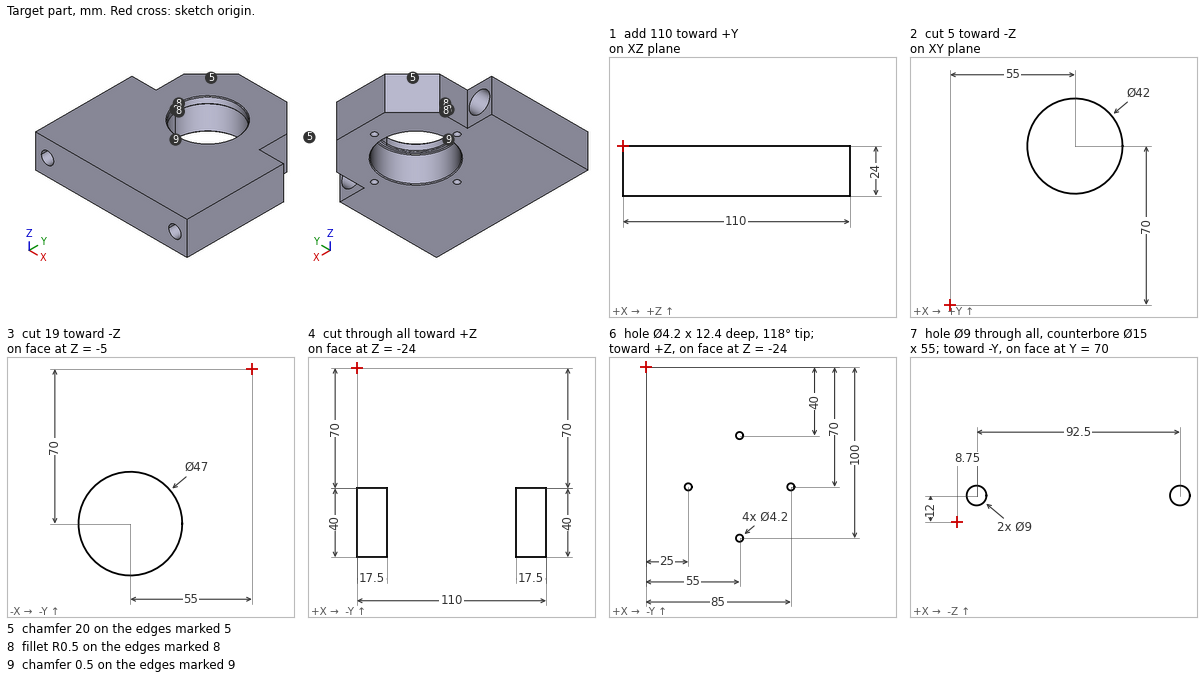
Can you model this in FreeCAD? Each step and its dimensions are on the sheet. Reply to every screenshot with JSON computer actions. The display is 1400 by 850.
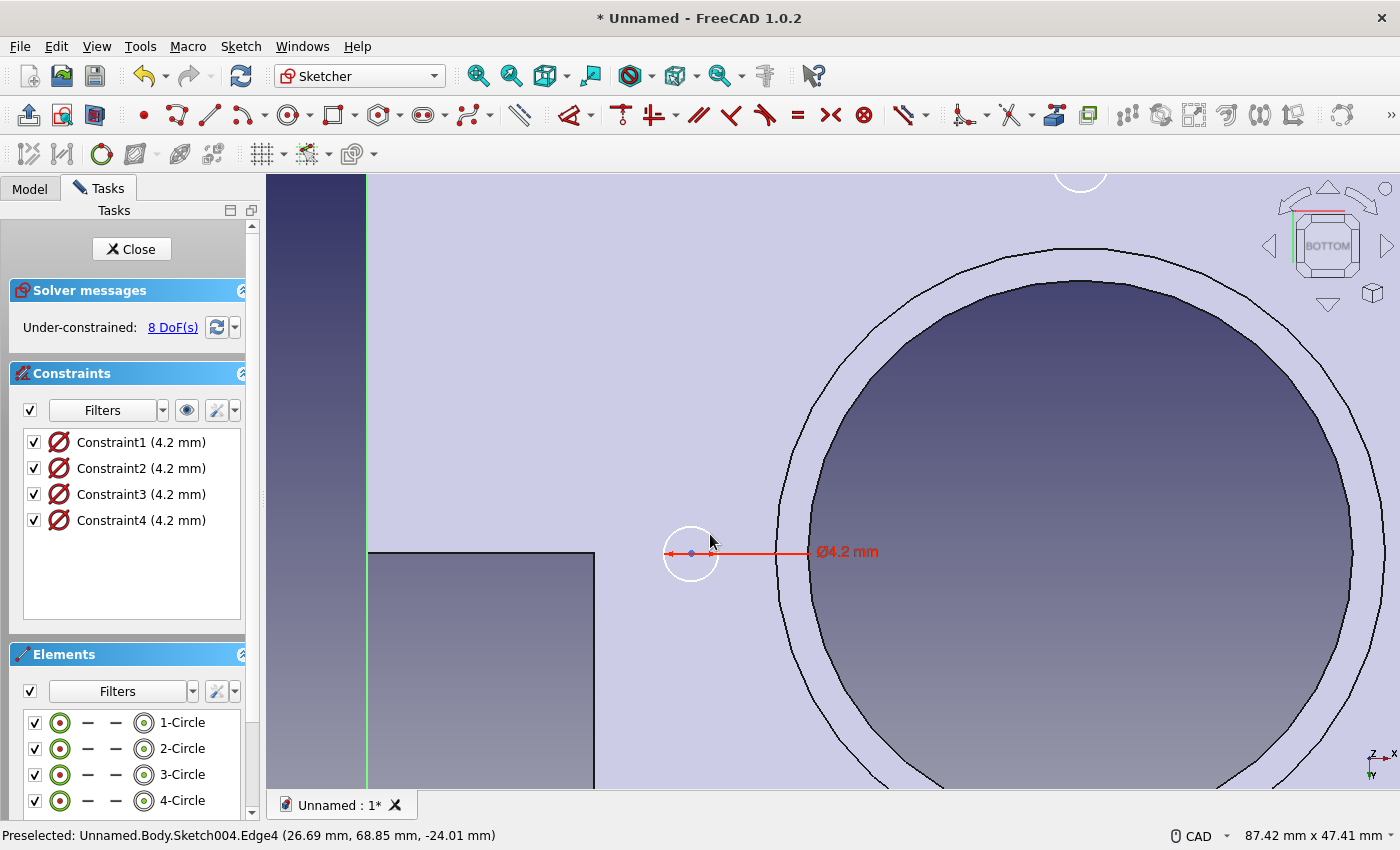
{"action": "scroll", "coordinate": [692, 557], "scroll_direction": "down", "scroll_amount": 6}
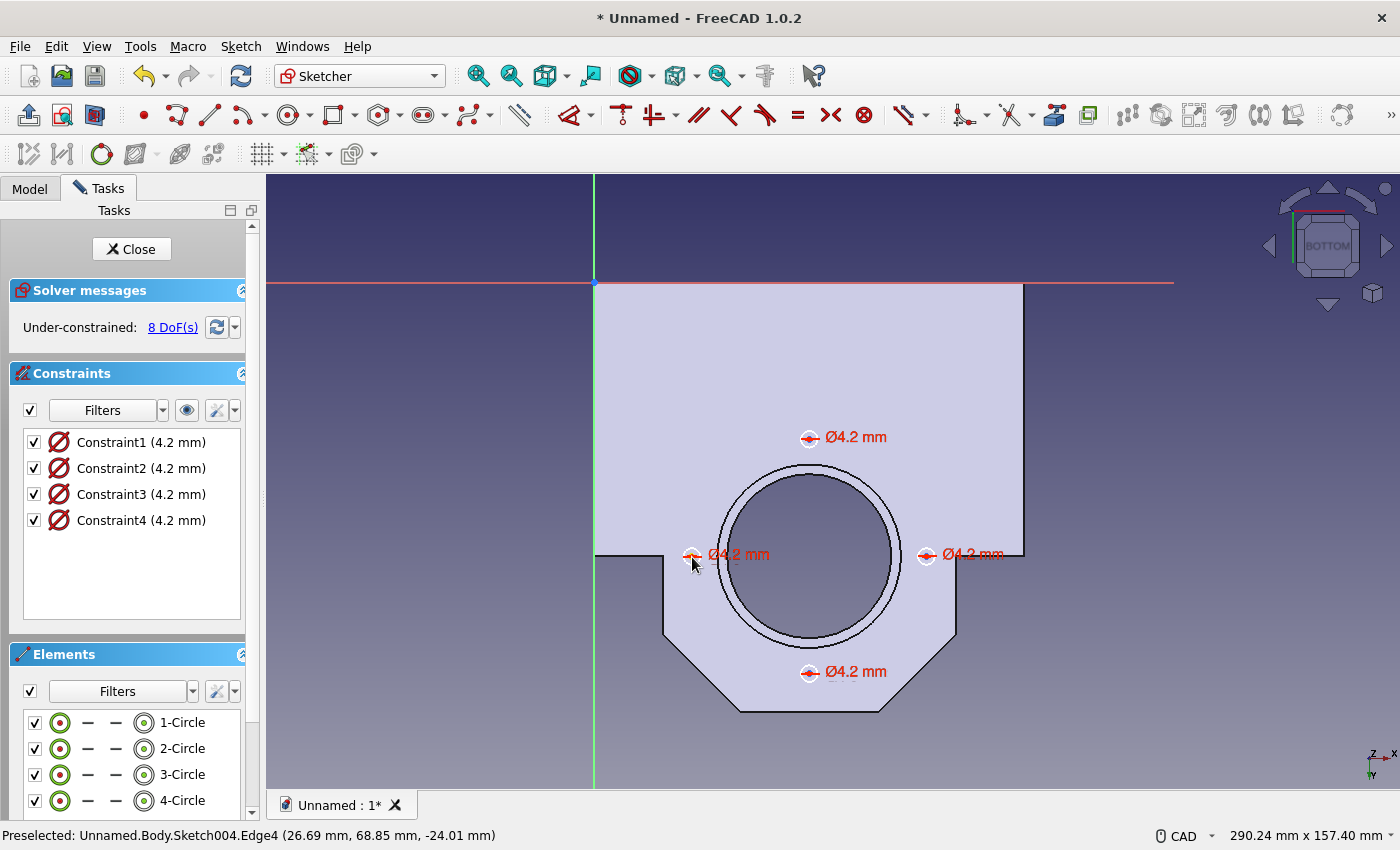
{"action": "left_click", "coordinate": [809, 674]}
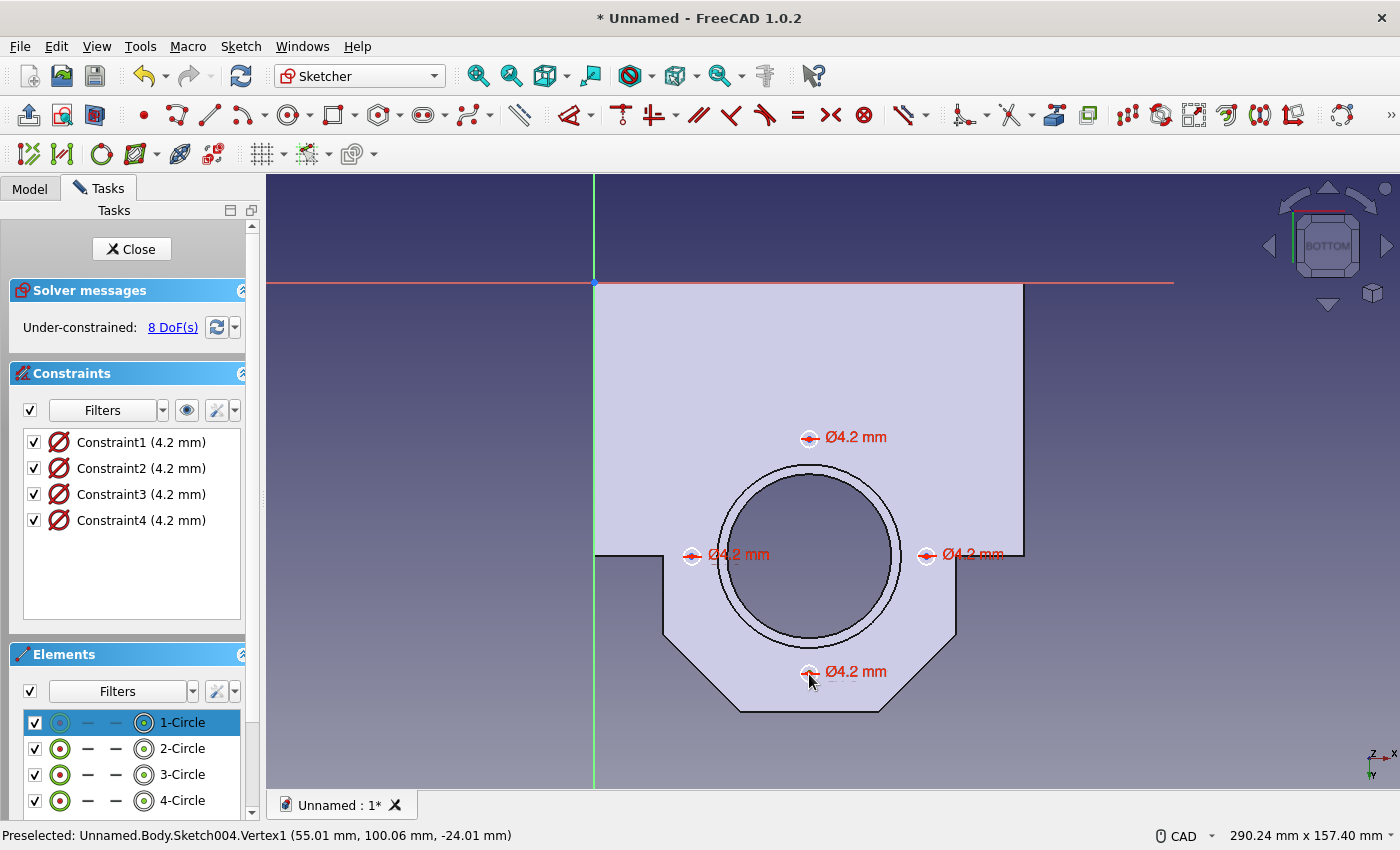
{"action": "left_click", "coordinate": [809, 439]}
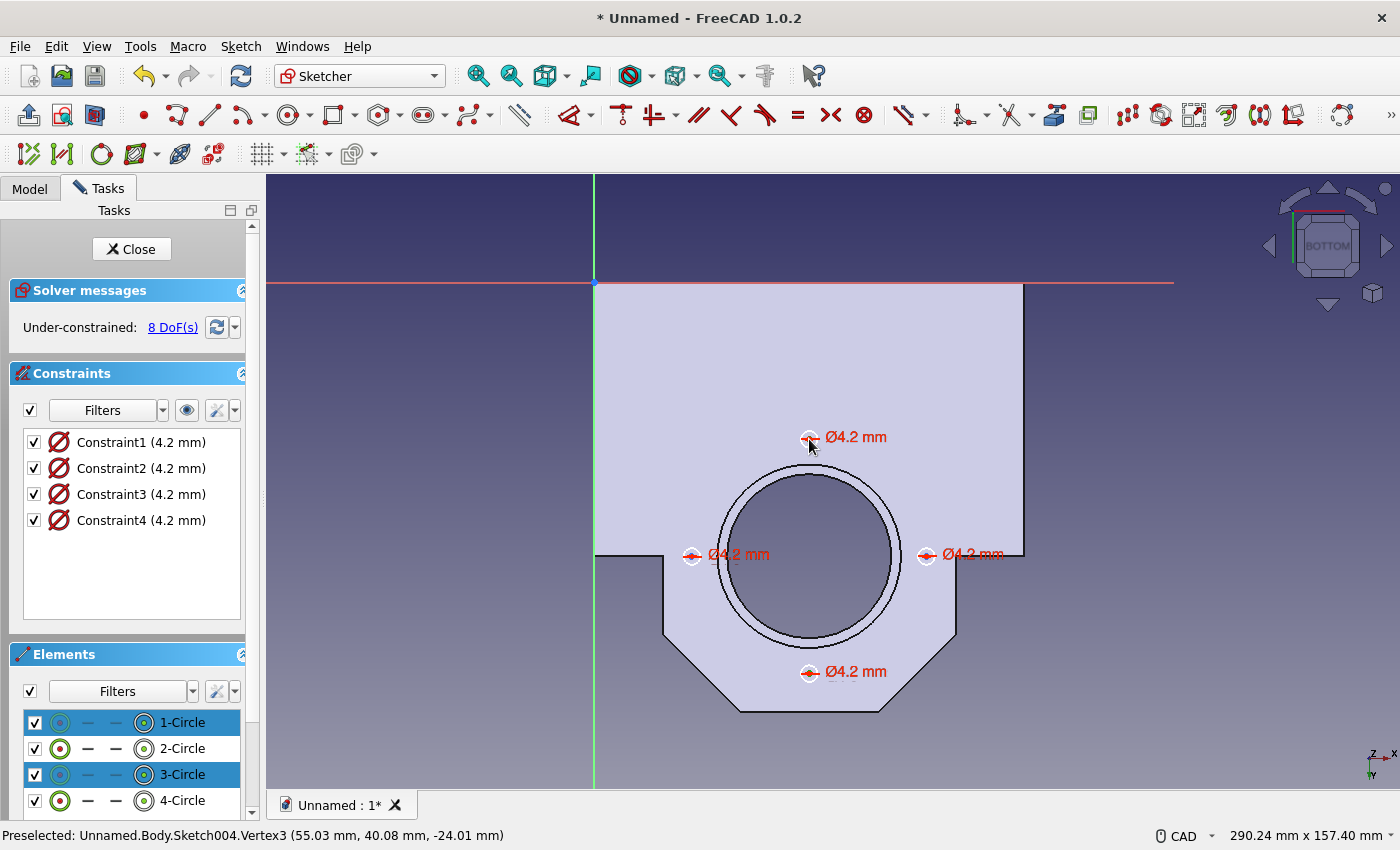
{"action": "key", "text": "v"}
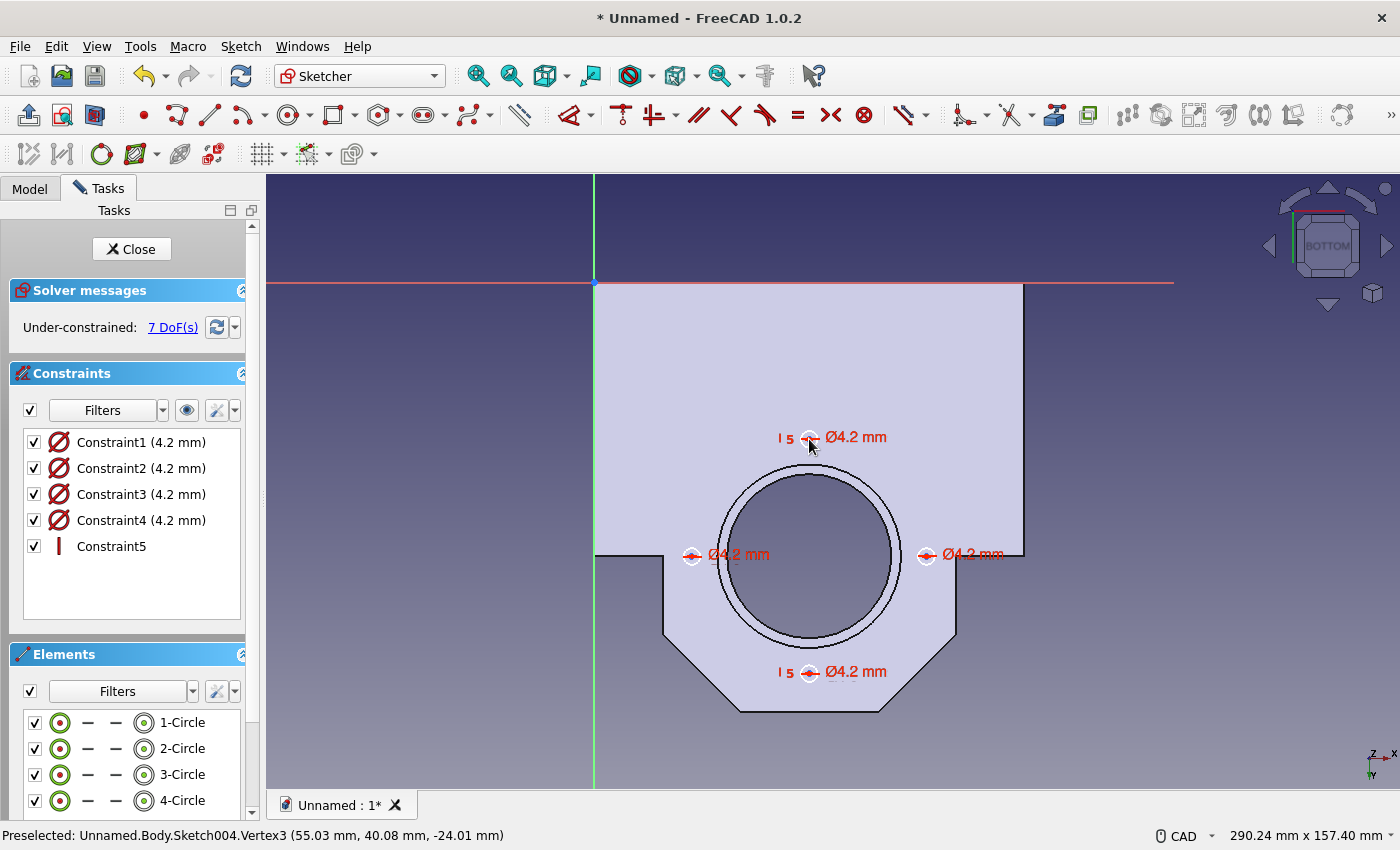
{"action": "left_click", "coordinate": [926, 556]}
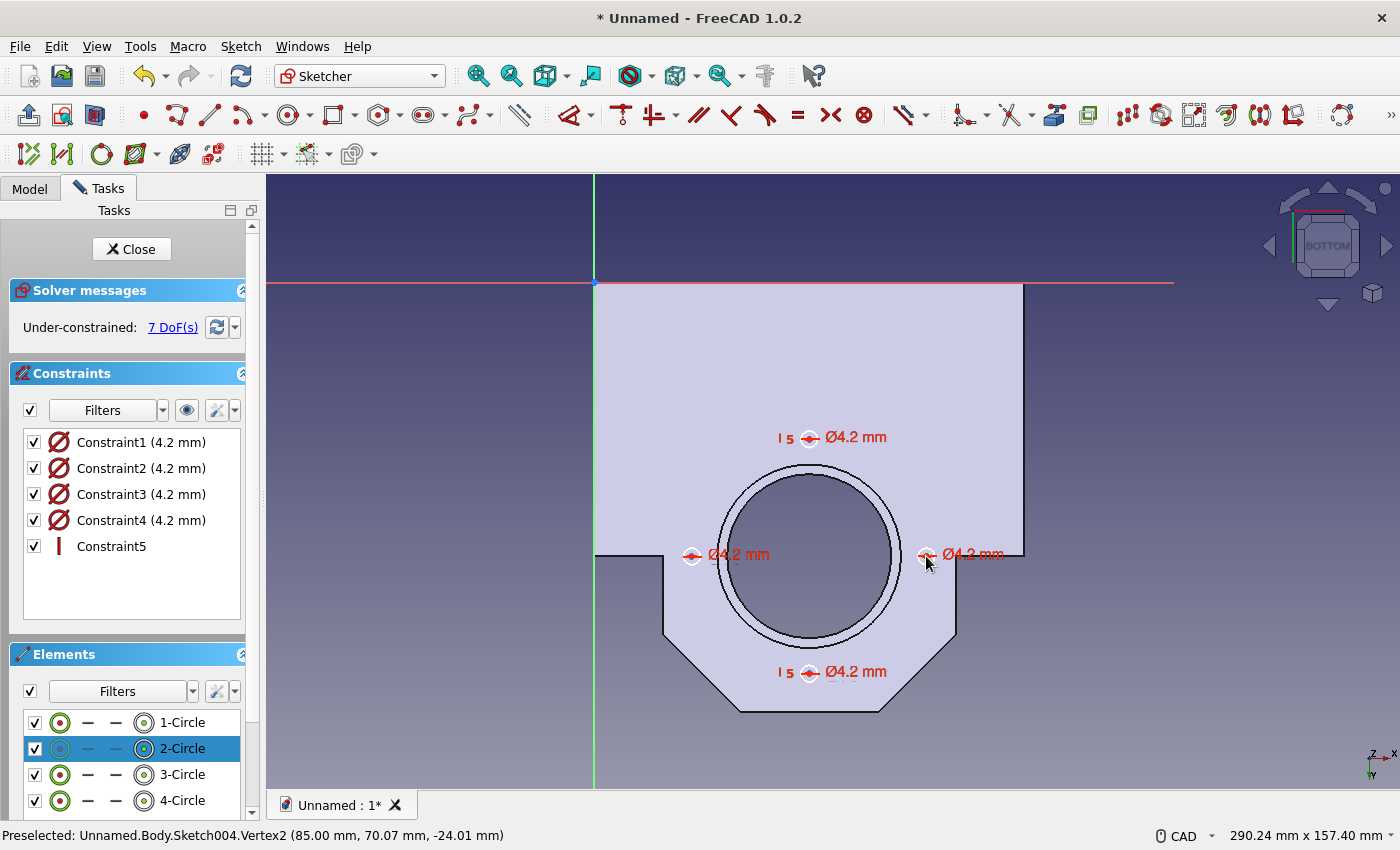
{"action": "left_click", "coordinate": [692, 557]}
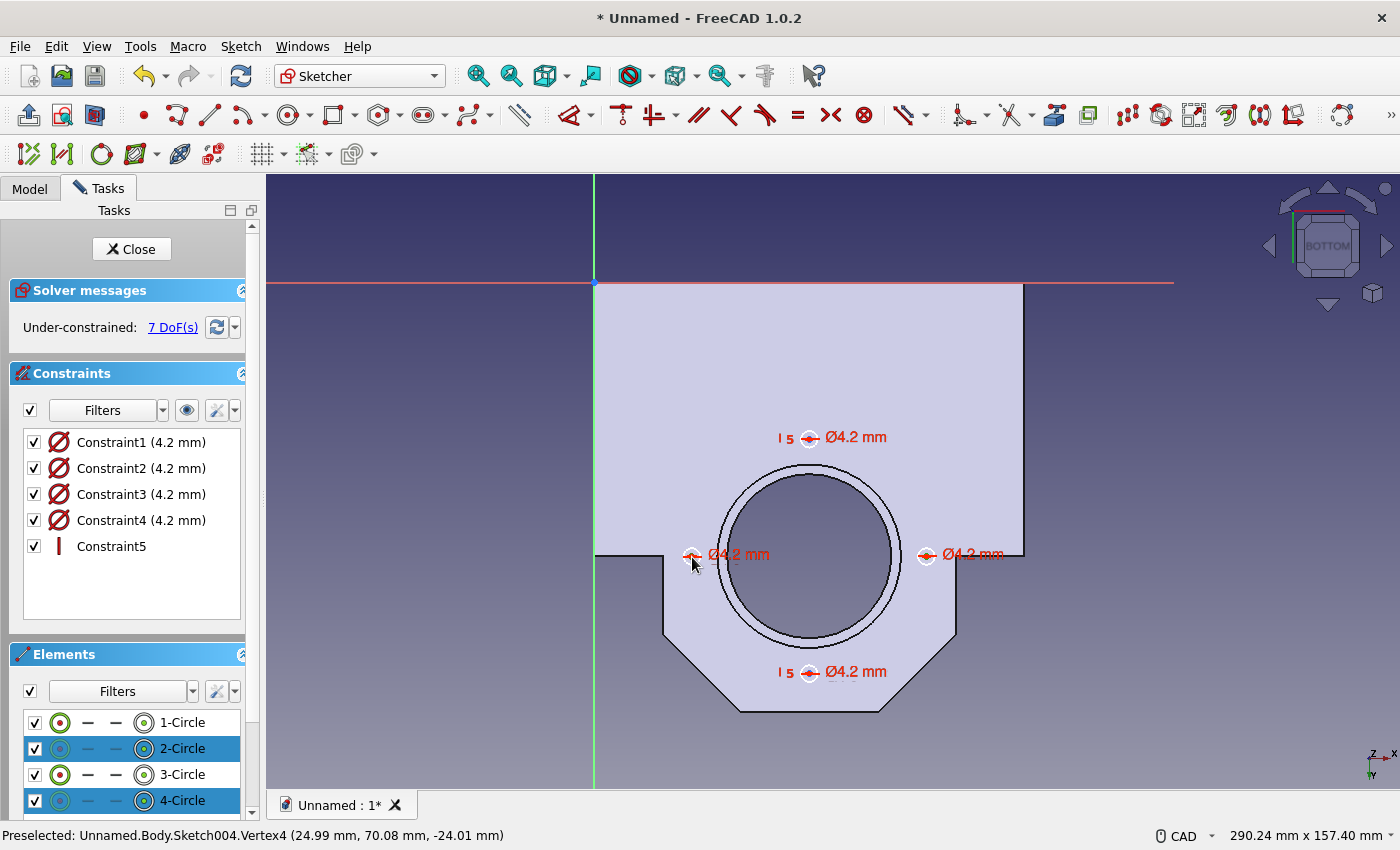
{"action": "left_click", "coordinate": [676, 116]}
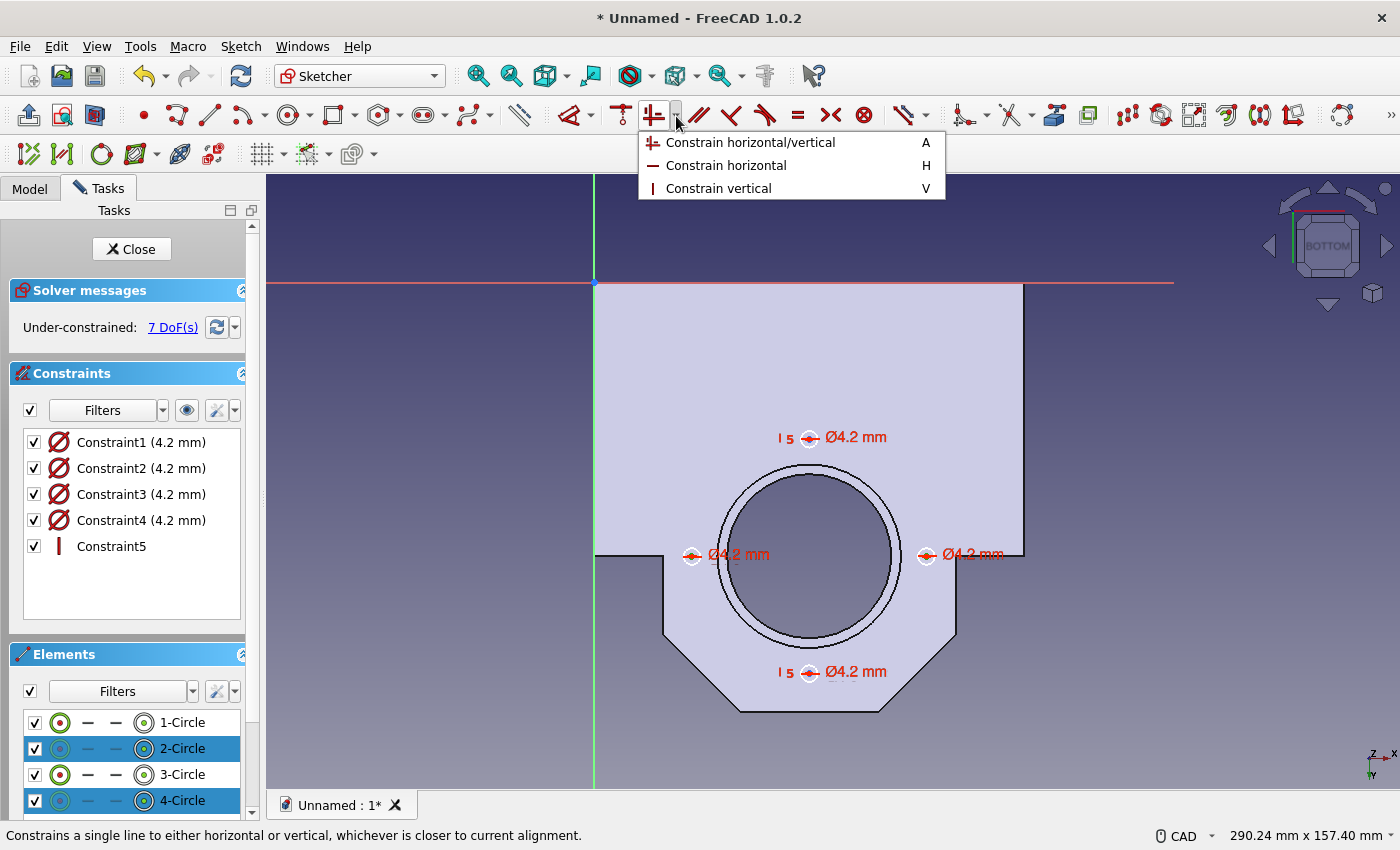
{"action": "left_click", "coordinate": [792, 166]}